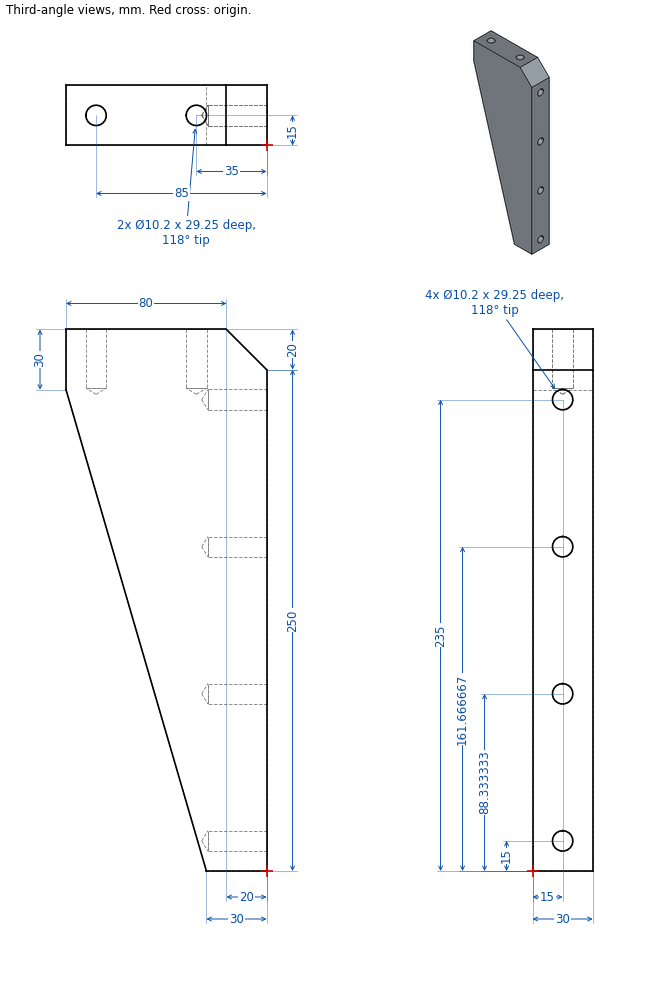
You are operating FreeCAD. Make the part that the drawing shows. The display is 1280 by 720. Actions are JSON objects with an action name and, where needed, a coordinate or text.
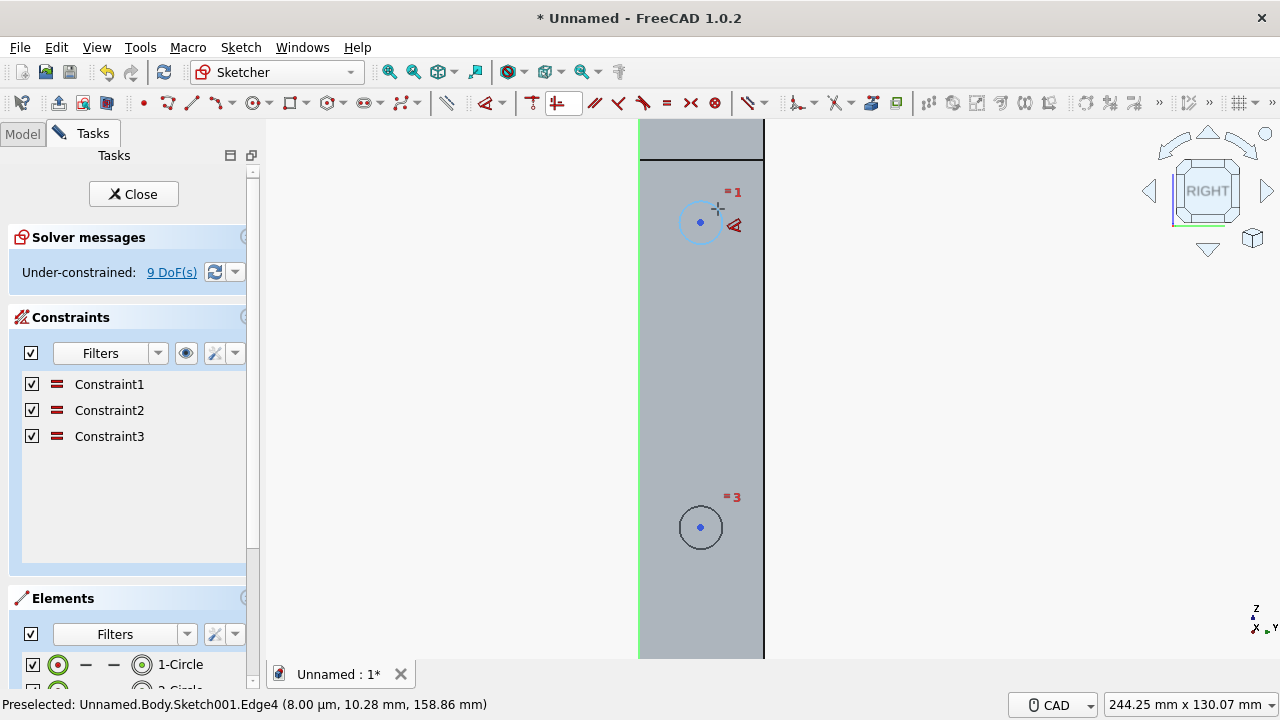
{"action": "left_click", "coordinate": [716, 208]}
{"action": "left_click", "coordinate": [739, 186]}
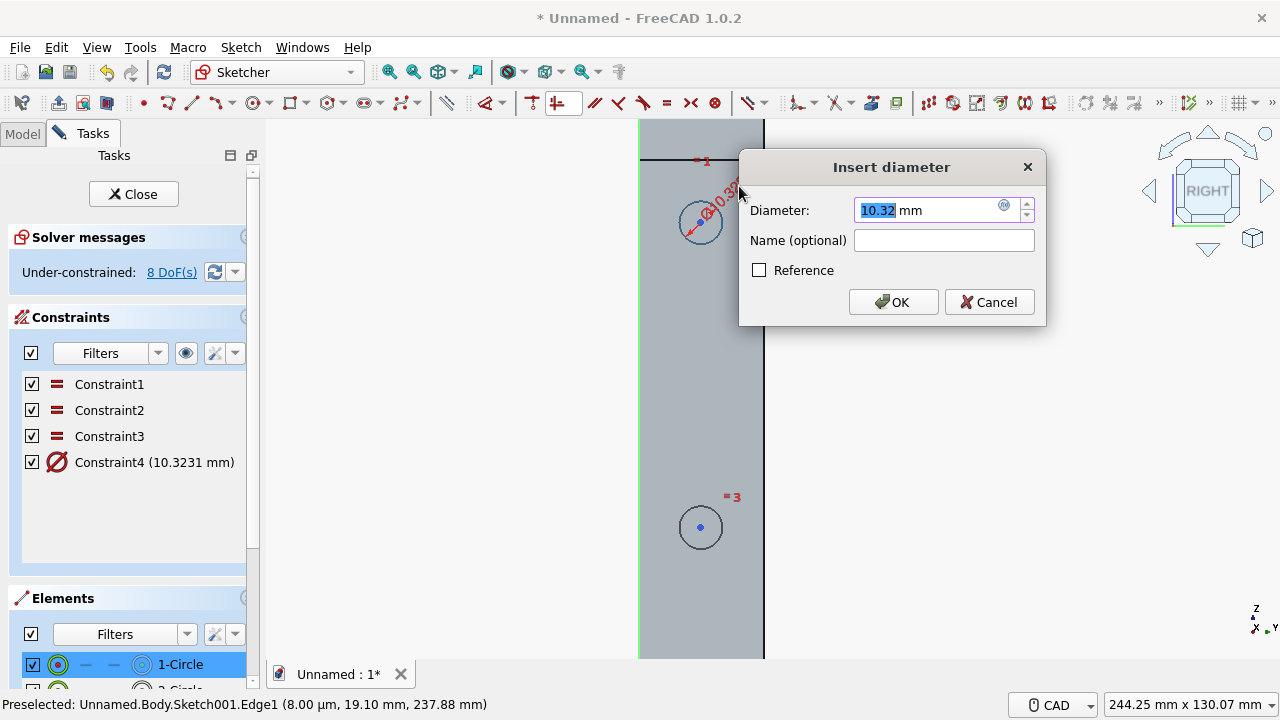
{"action": "type", "text": "10.2"}
{"action": "key", "text": "Return"}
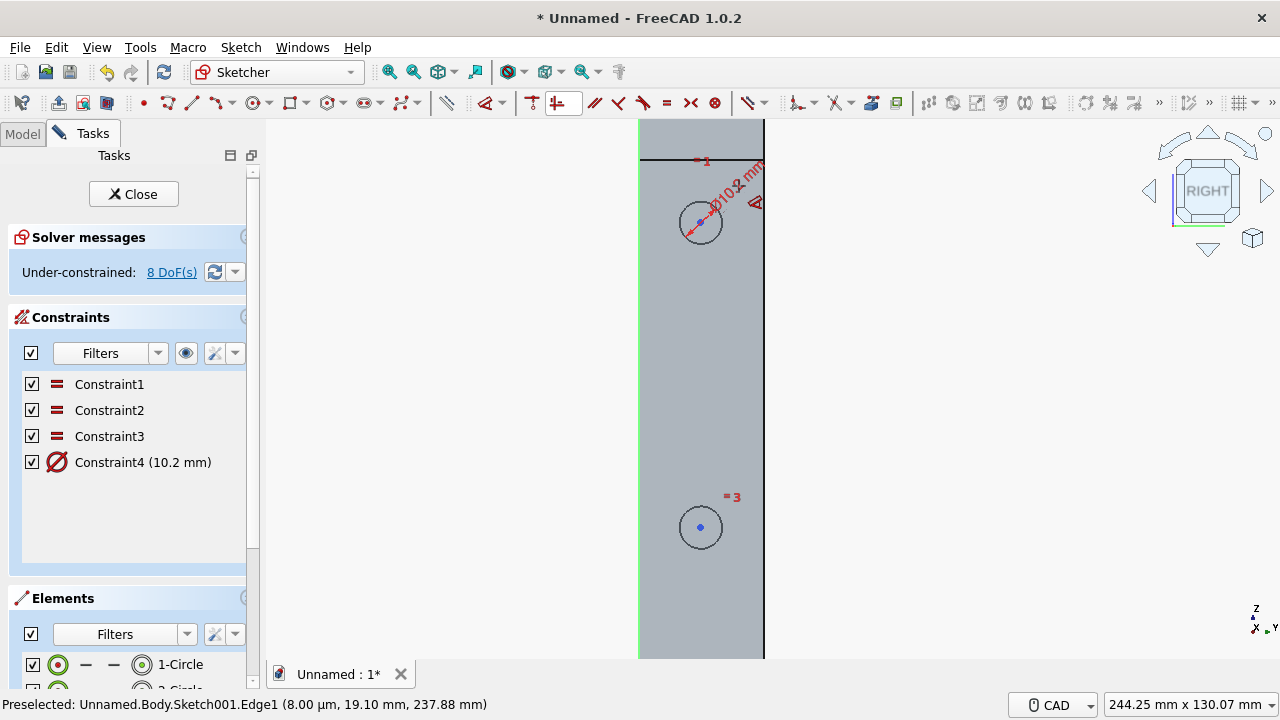
{"action": "left_click", "coordinate": [701, 223]}
{"action": "left_click", "coordinate": [656, 189]}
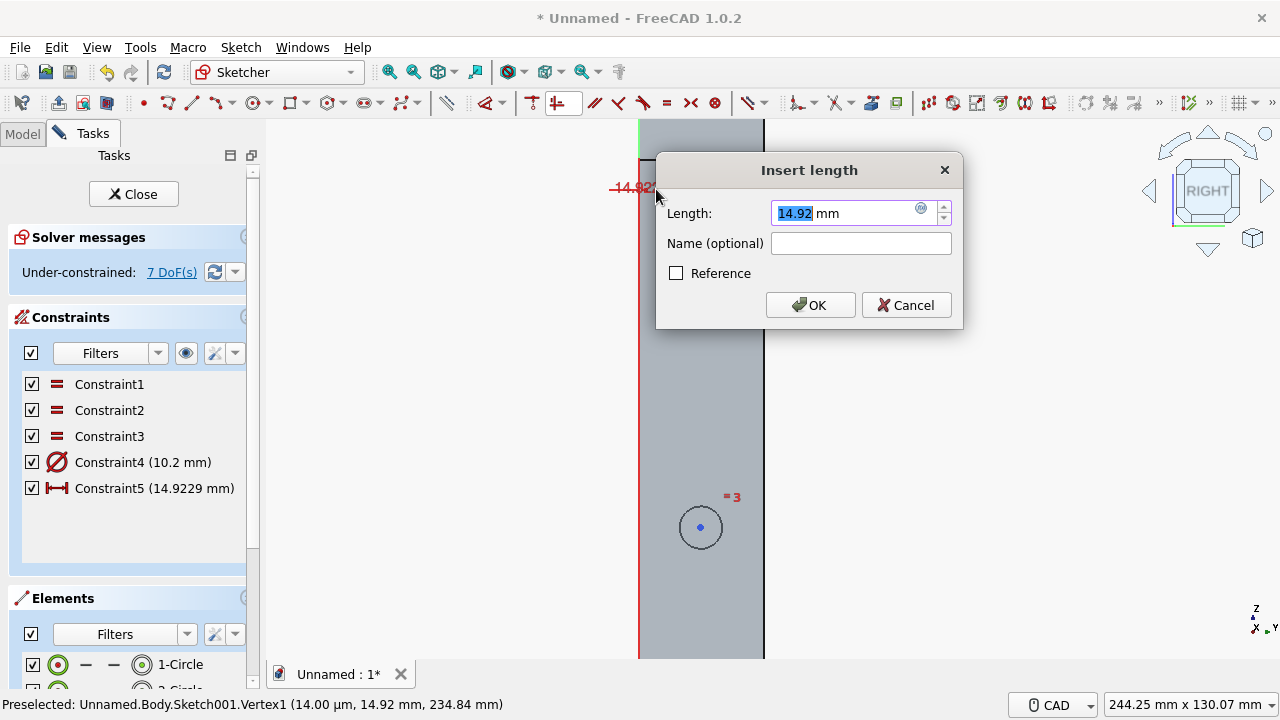
{"action": "type", "text": "15"}
{"action": "key", "text": "Return"}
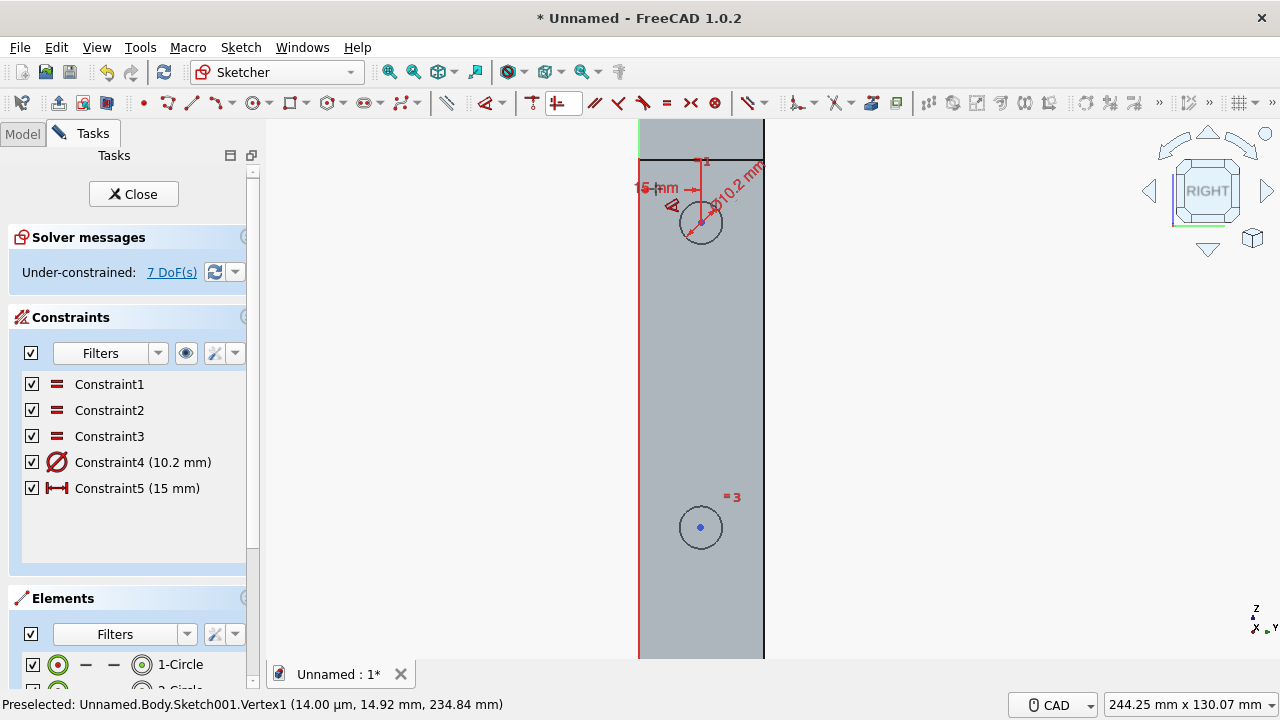
{"action": "scroll", "coordinate": [718, 208], "scroll_direction": "down", "scroll_amount": 5}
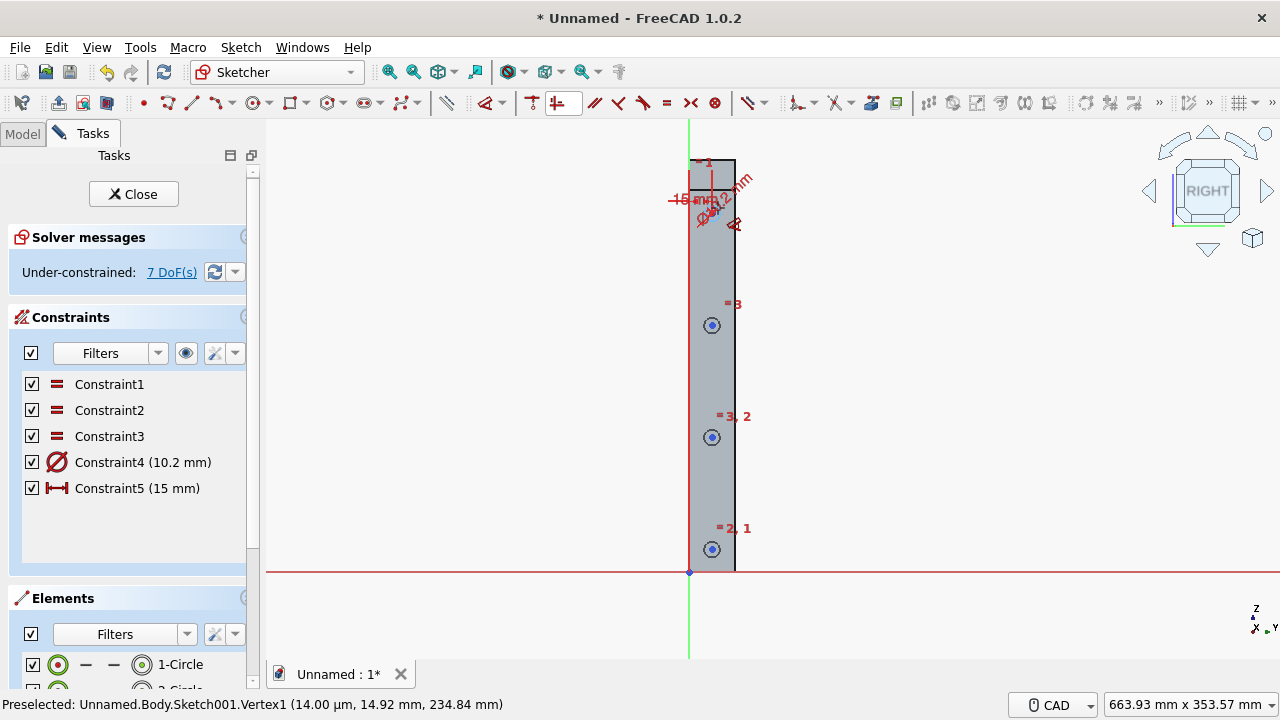
{"action": "scroll", "coordinate": [712, 550], "scroll_direction": "up", "scroll_amount": 3}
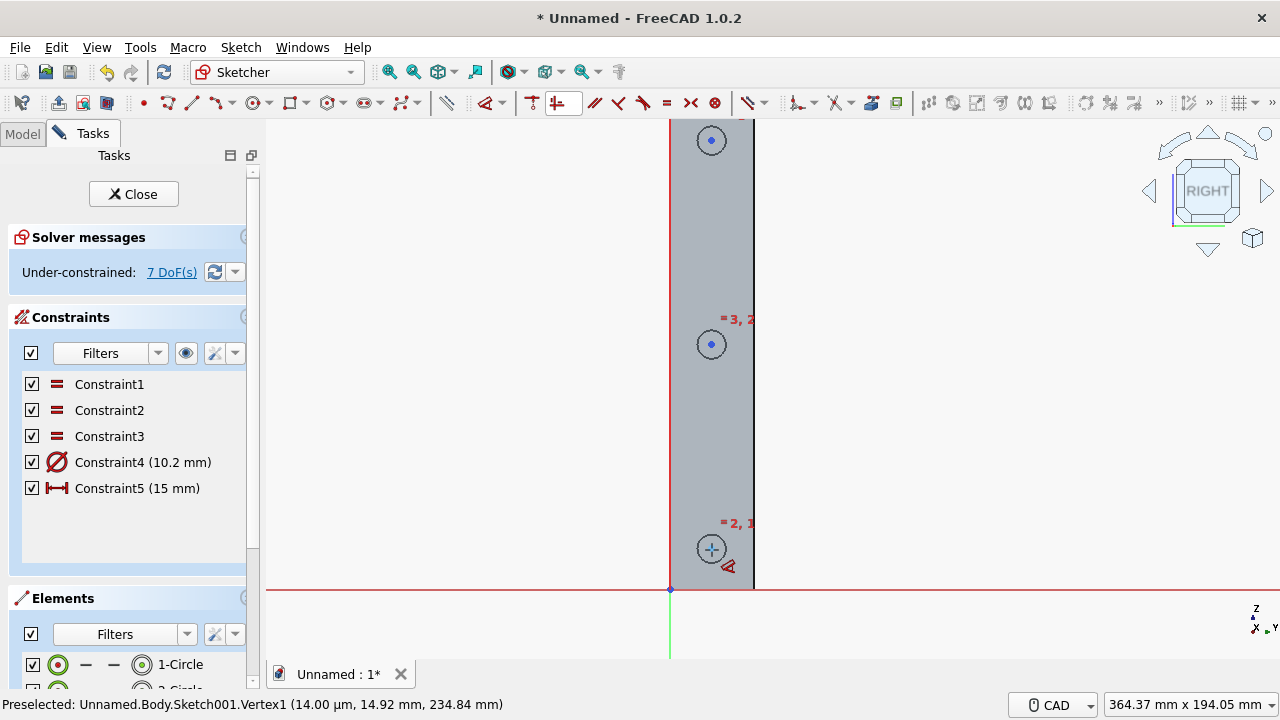
{"action": "left_click", "coordinate": [712, 549]}
{"action": "left_click", "coordinate": [691, 624]}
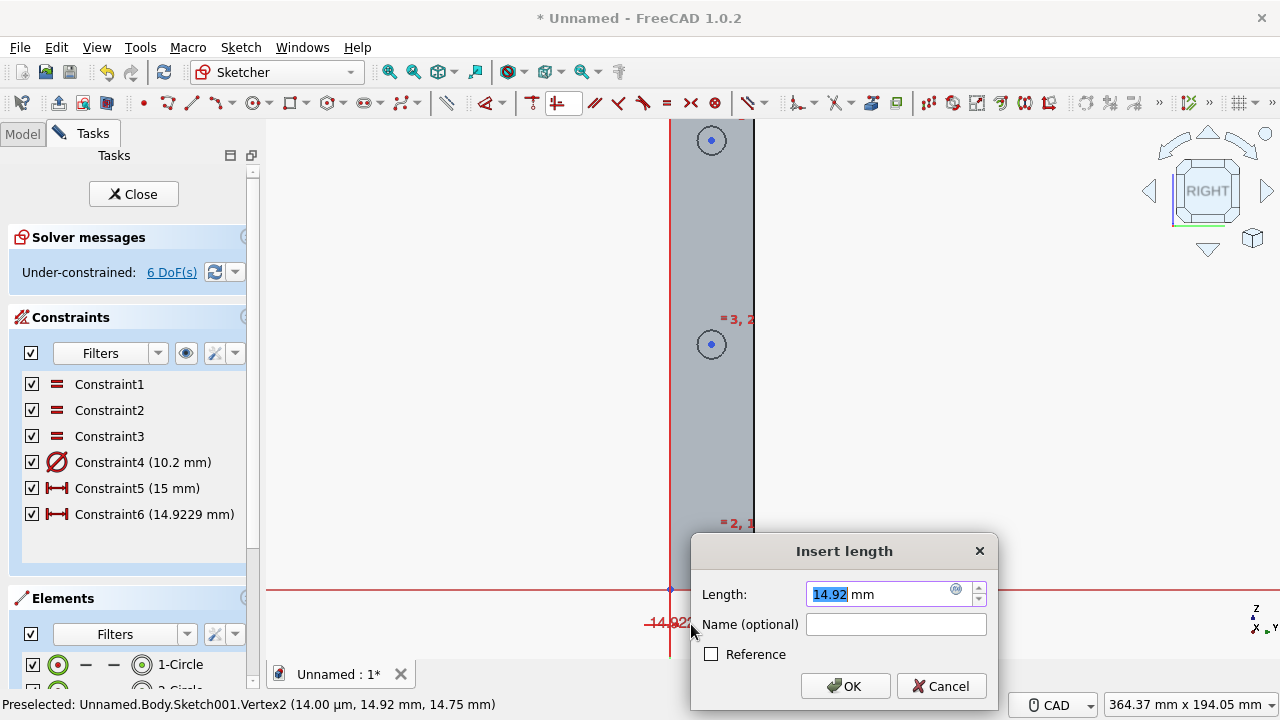
{"action": "type", "text": "15"}
{"action": "key", "text": "Return"}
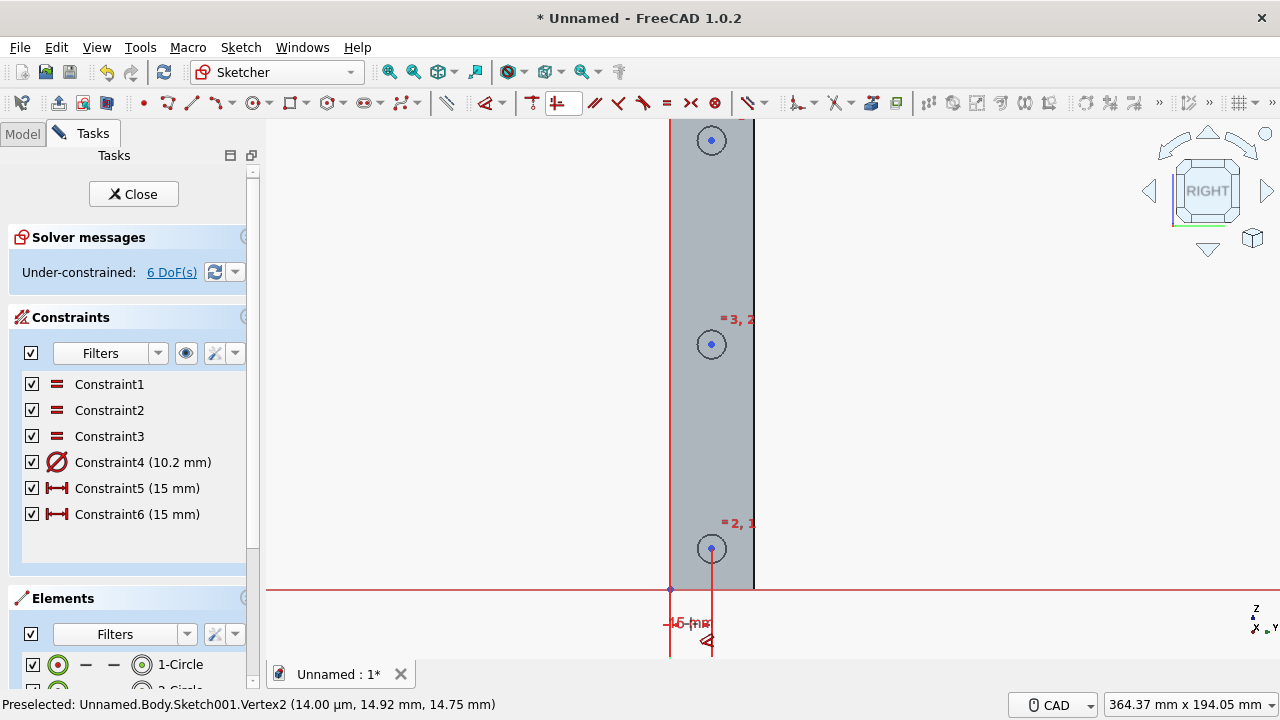
{"action": "left_click", "coordinate": [712, 549]}
{"action": "left_click", "coordinate": [636, 569]}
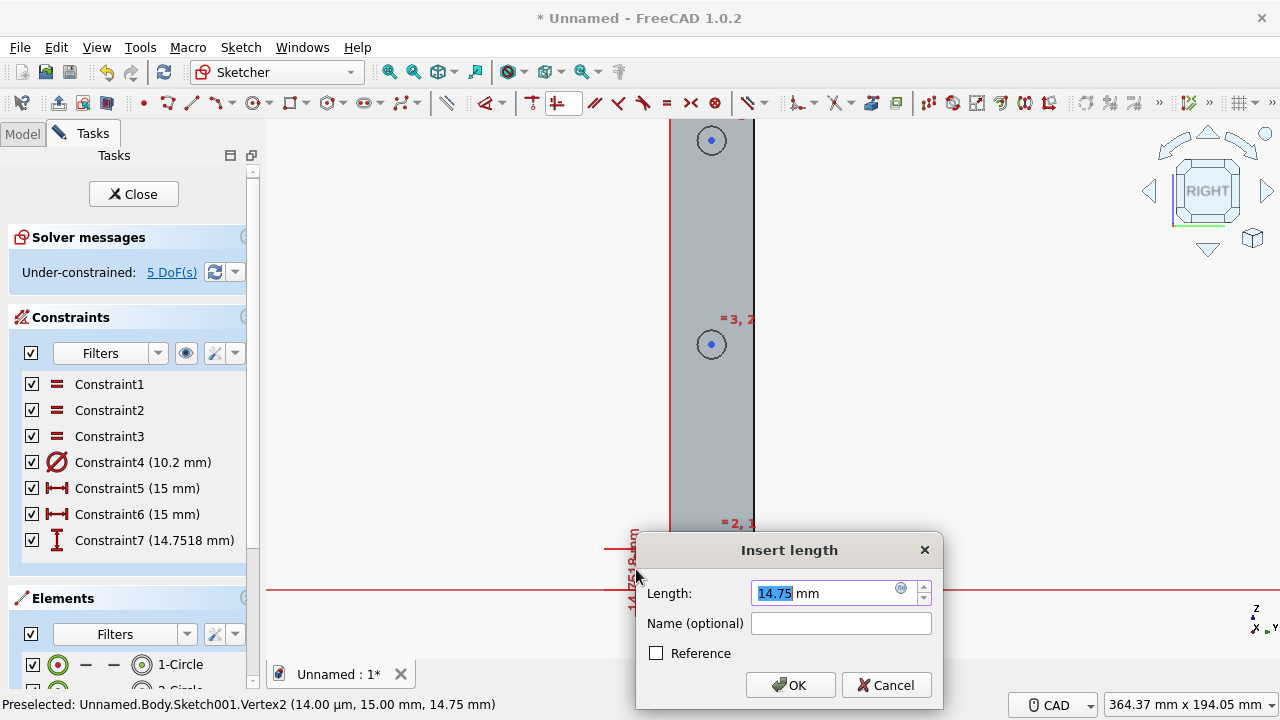
{"action": "type", "text": "15"}
{"action": "key", "text": "Return"}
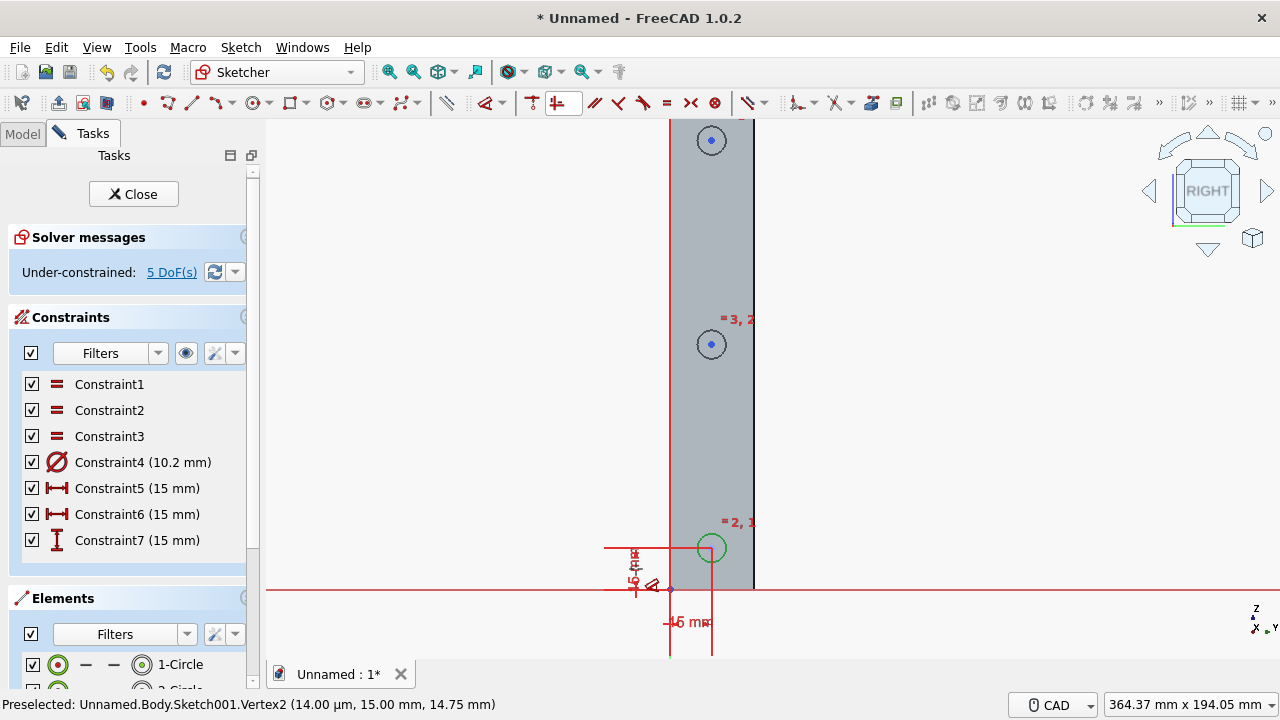
{"action": "left_click", "coordinate": [712, 345]}
{"action": "left_click", "coordinate": [691, 311]}